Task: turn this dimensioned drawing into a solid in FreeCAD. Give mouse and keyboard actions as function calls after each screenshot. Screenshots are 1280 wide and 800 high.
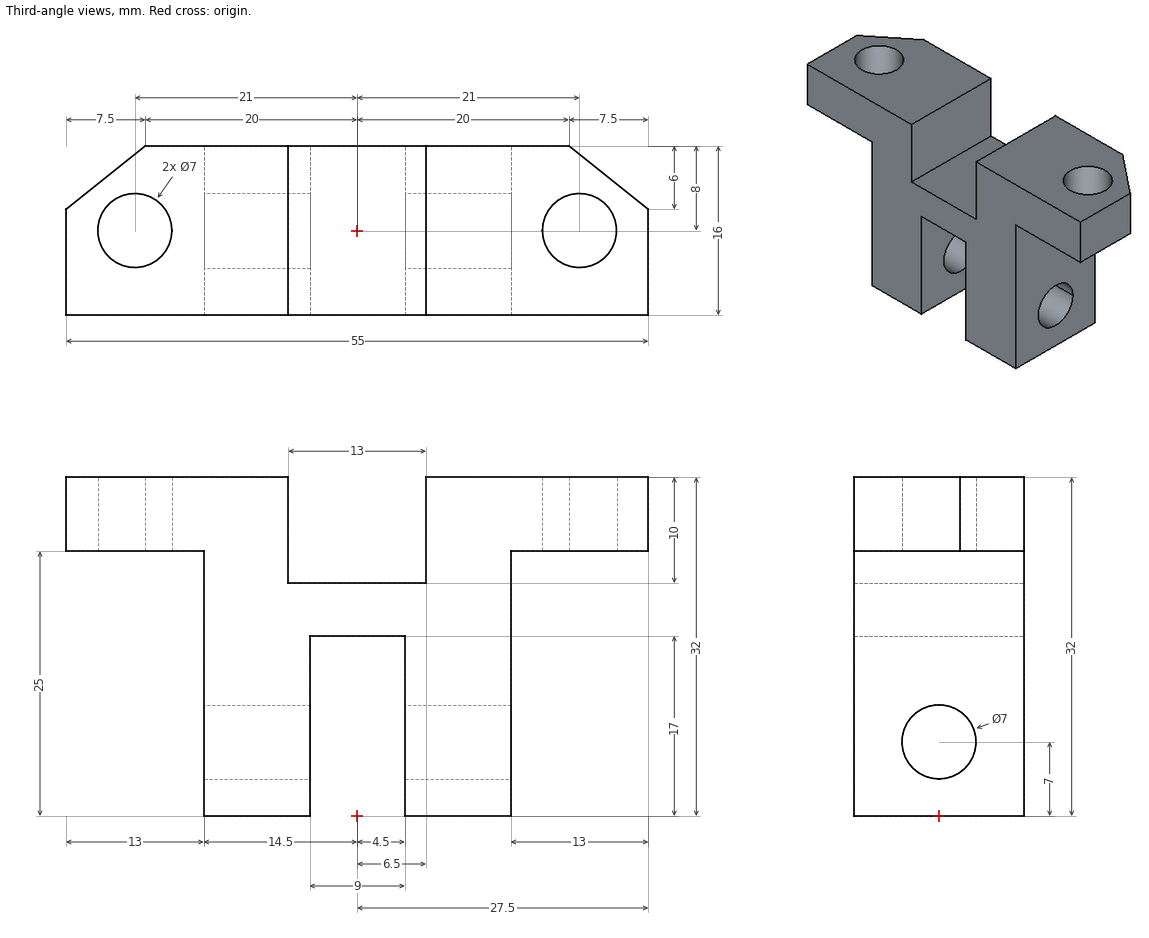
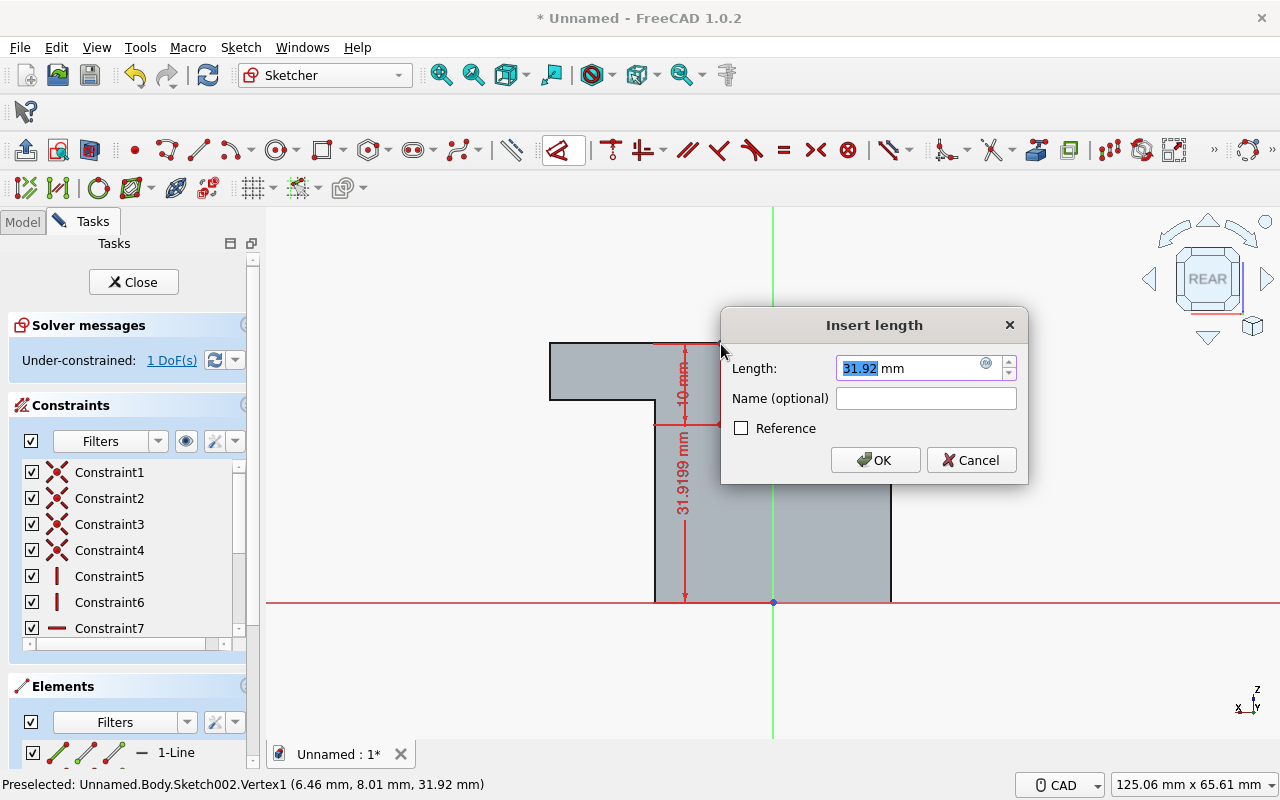
text(32)
key(Return)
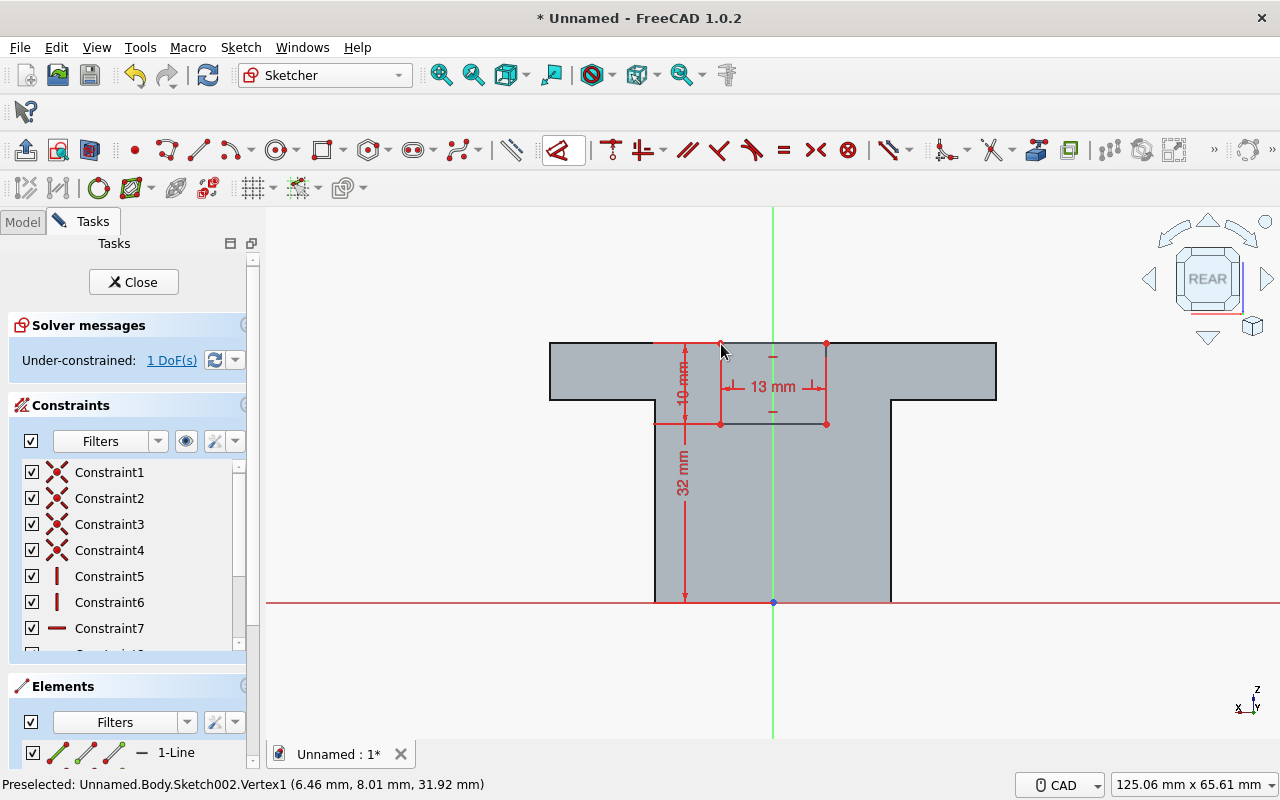
click(721, 343)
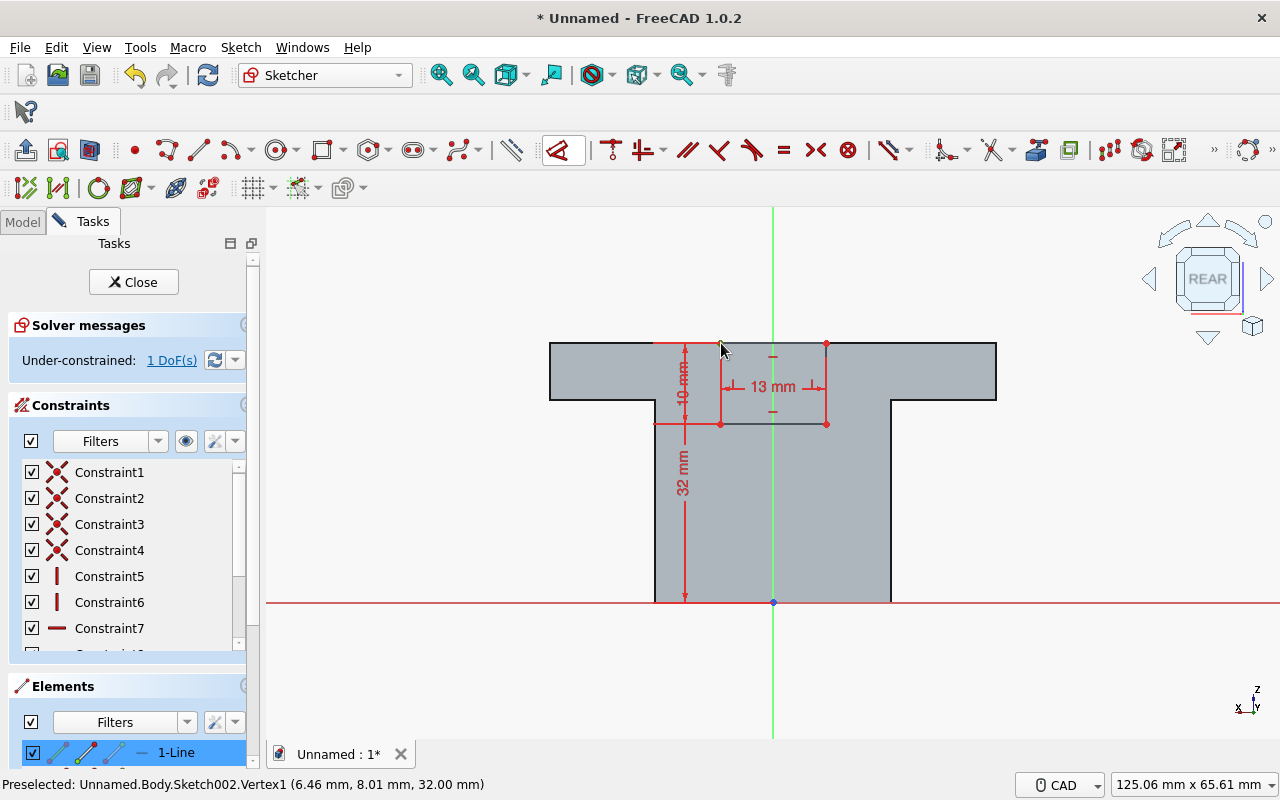
click(580, 150)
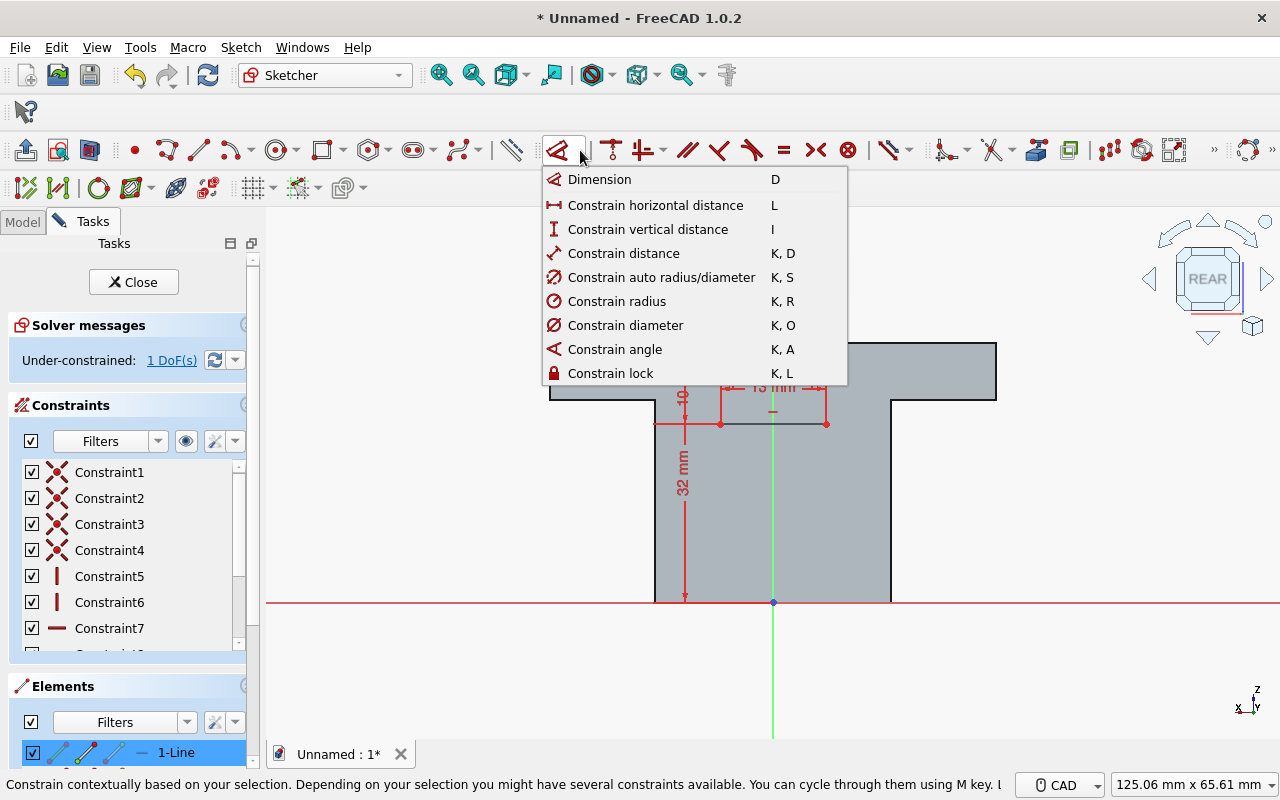
click(695, 205)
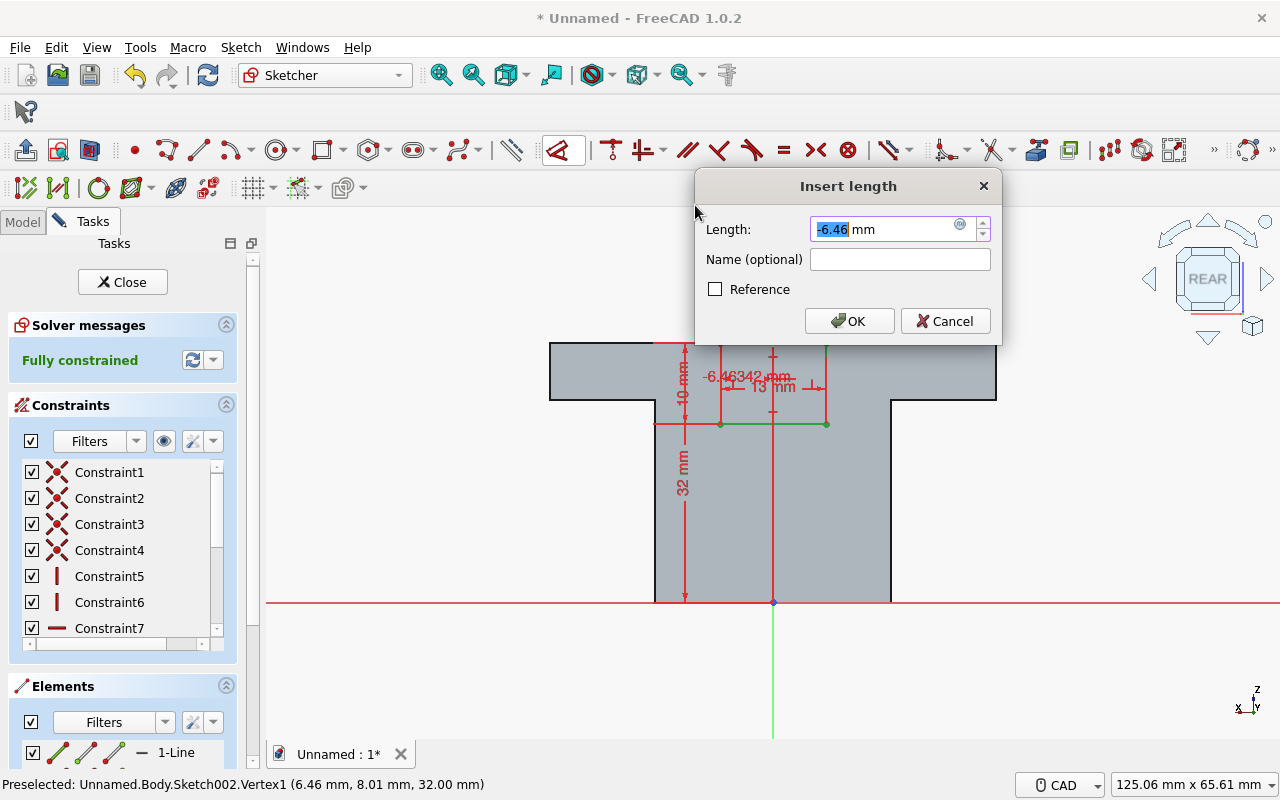
text(-6.5)
key(Return)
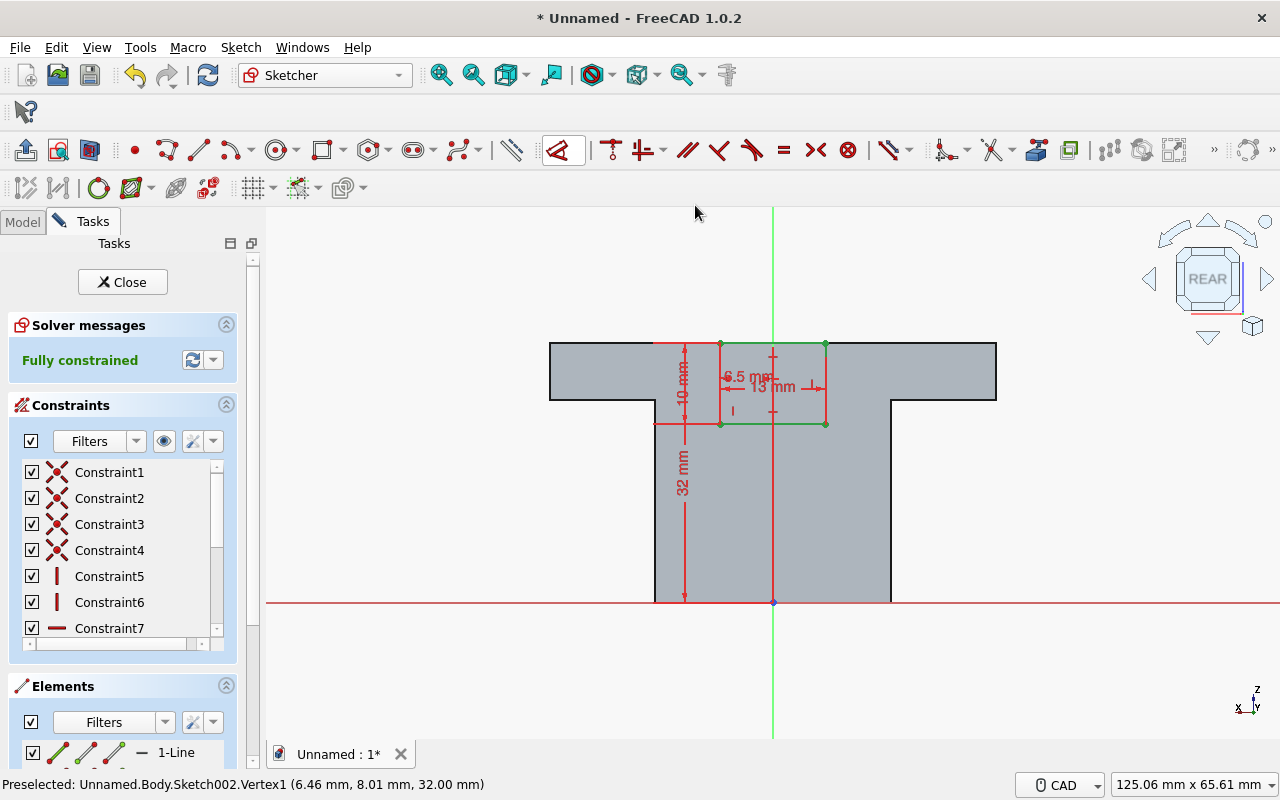
click(123, 282)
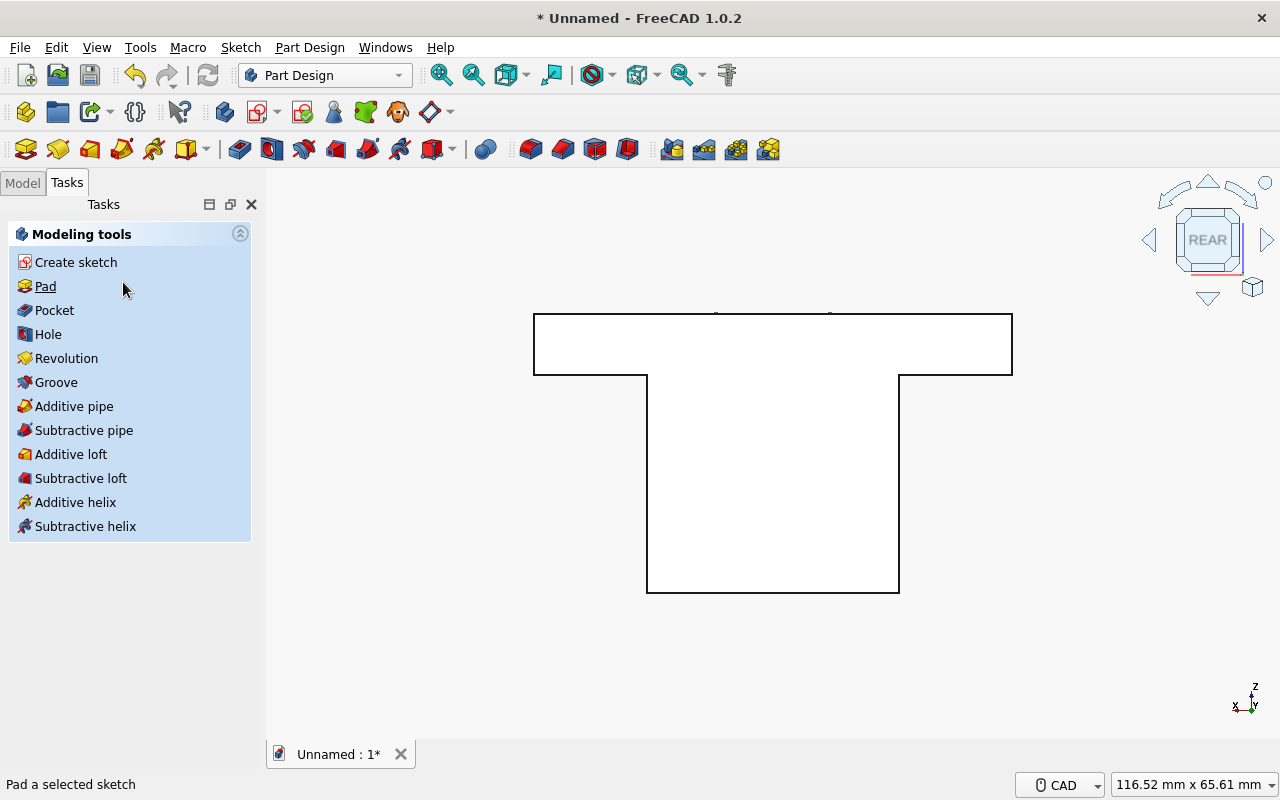
click(240, 150)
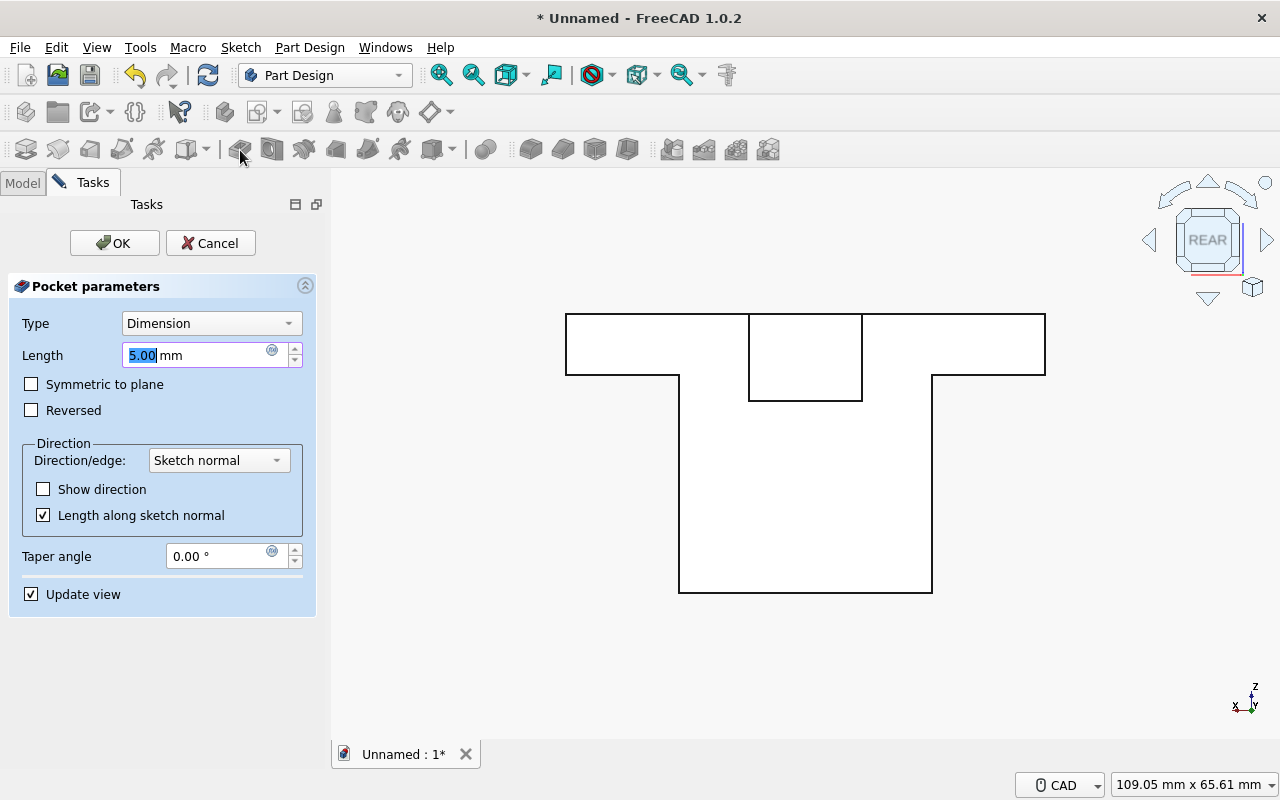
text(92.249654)
key(Tab)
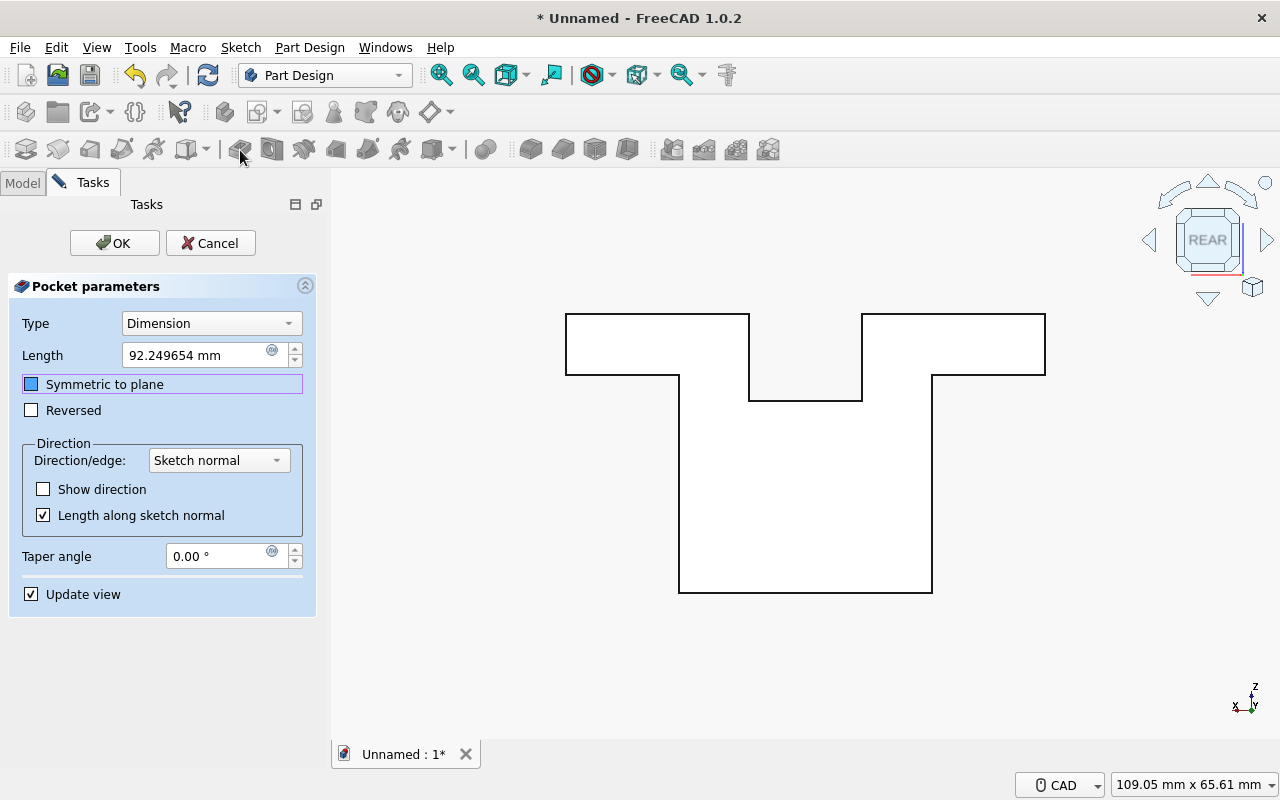
click(30, 384)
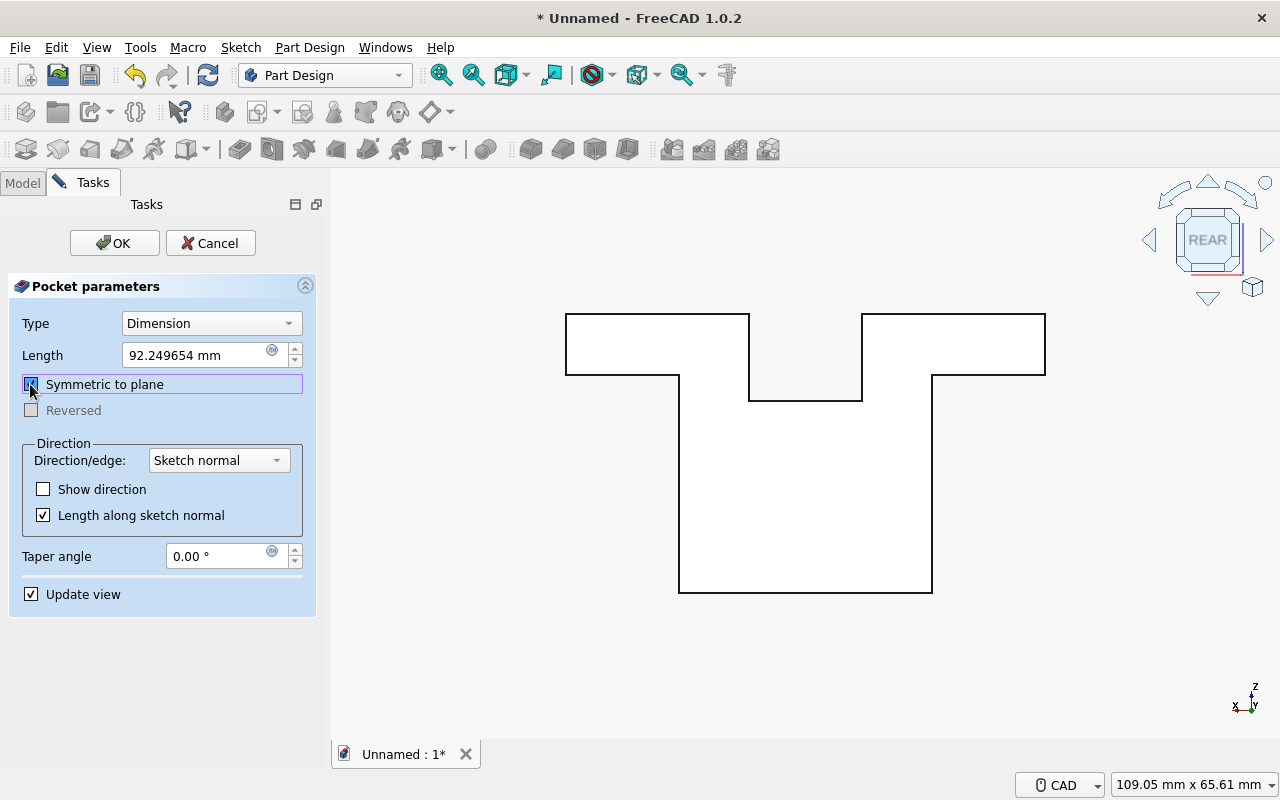
click(115, 243)